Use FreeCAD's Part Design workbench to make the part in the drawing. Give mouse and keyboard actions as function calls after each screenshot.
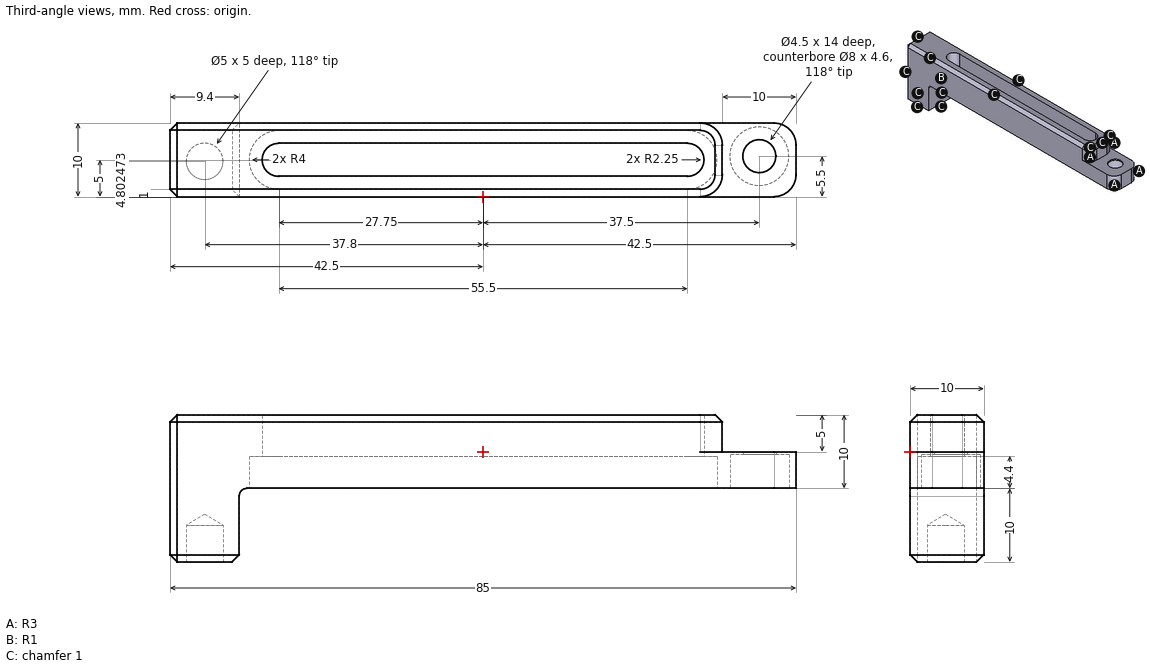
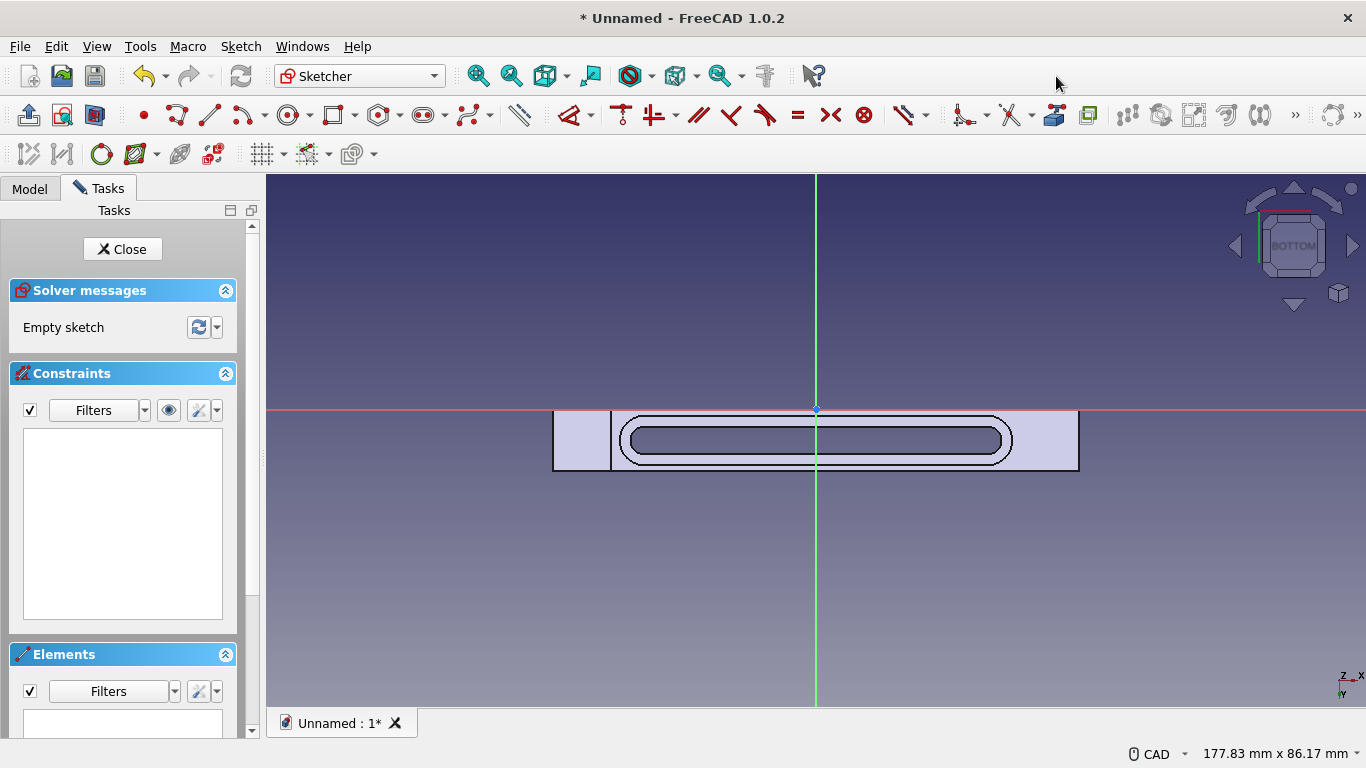
scroll(566, 439, up, 12)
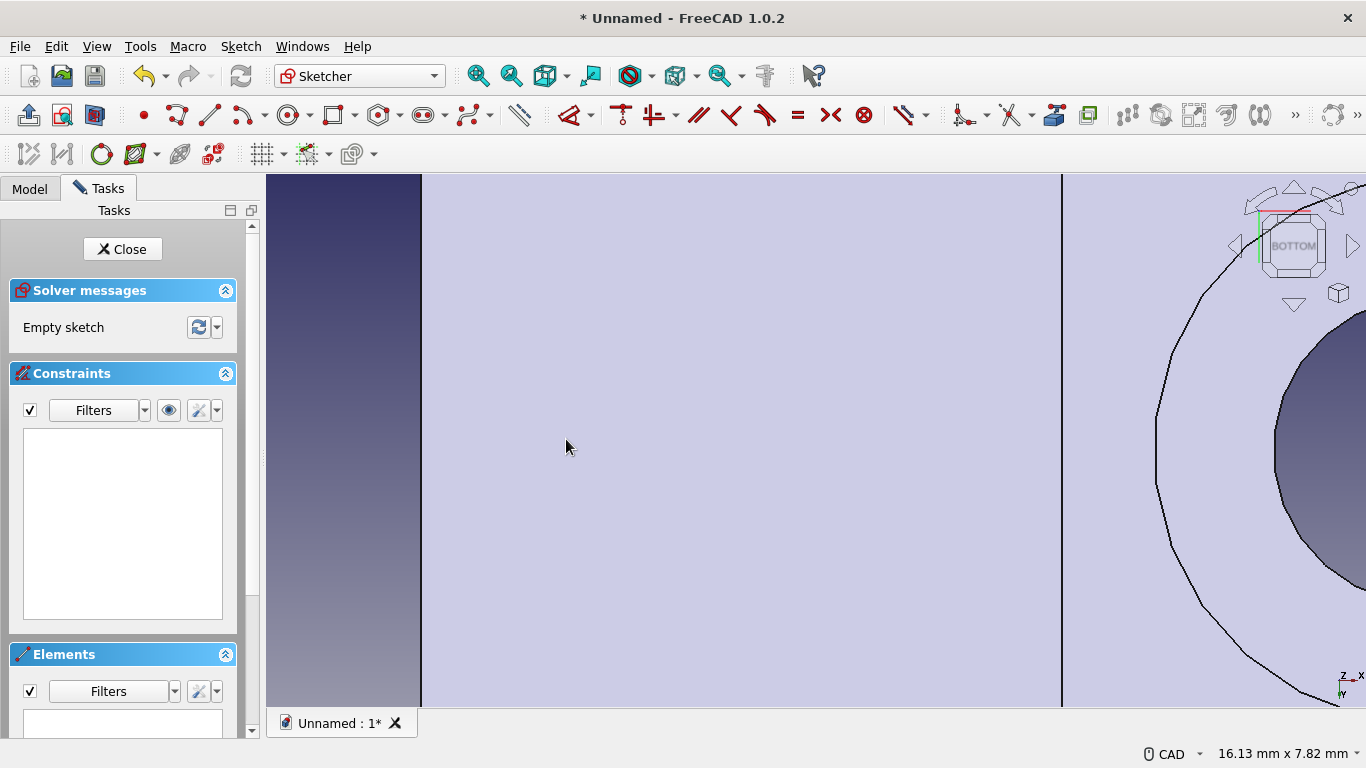
key(g)
key(c)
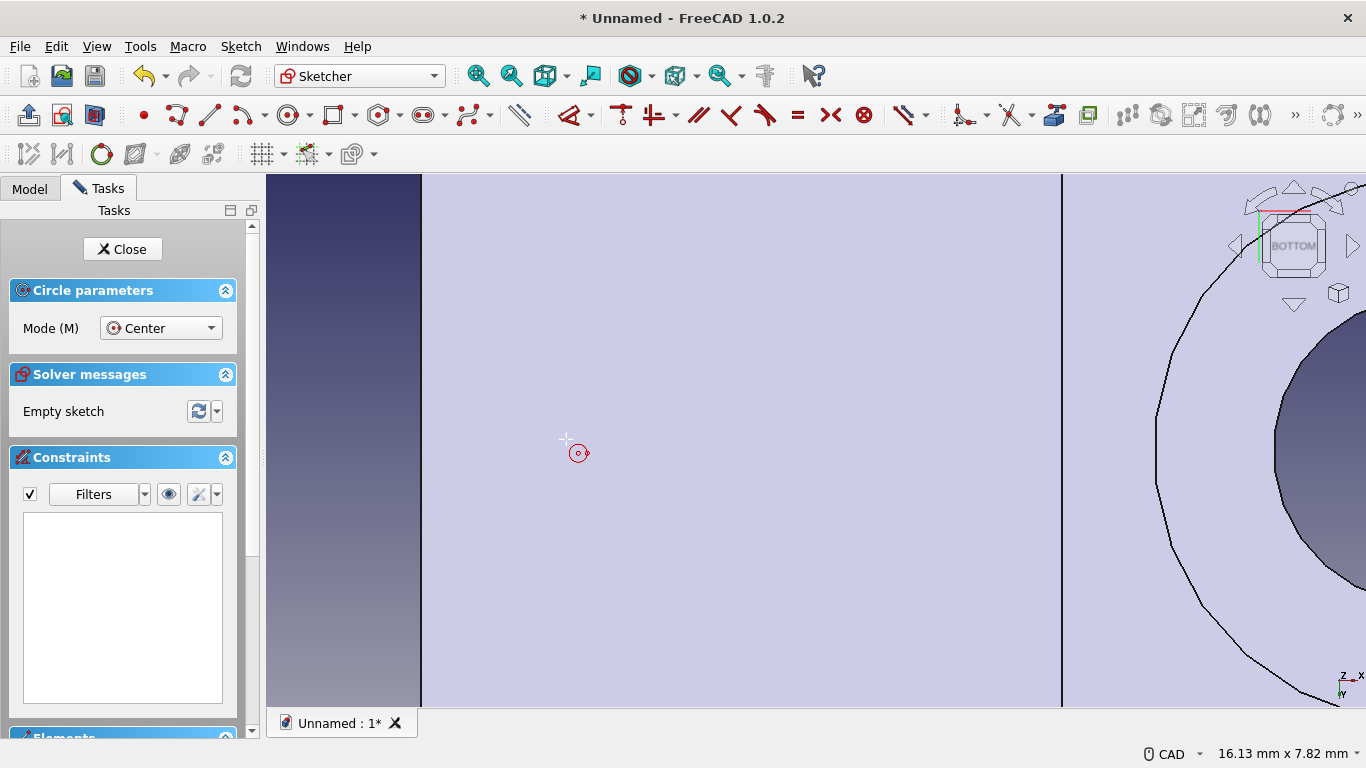
click(742, 437)
click(862, 317)
key(Escape)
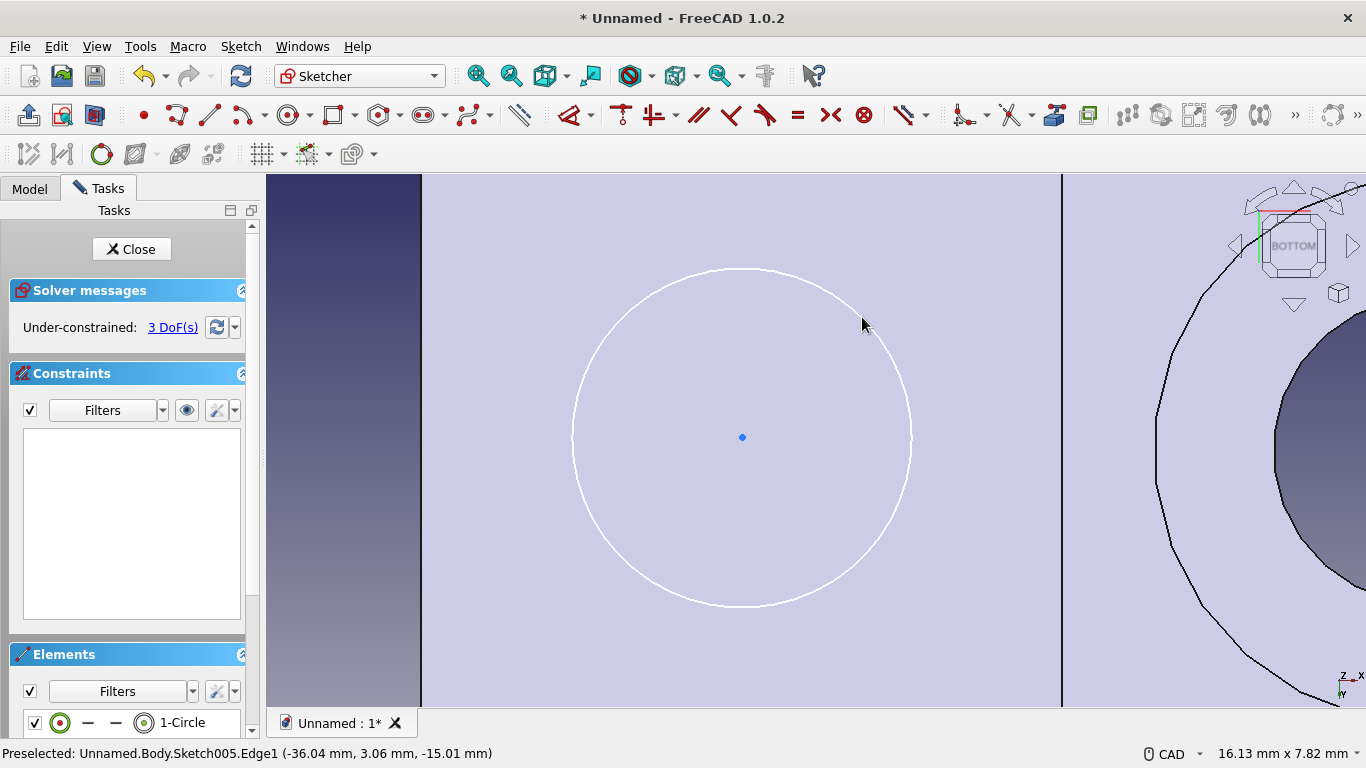
key(d)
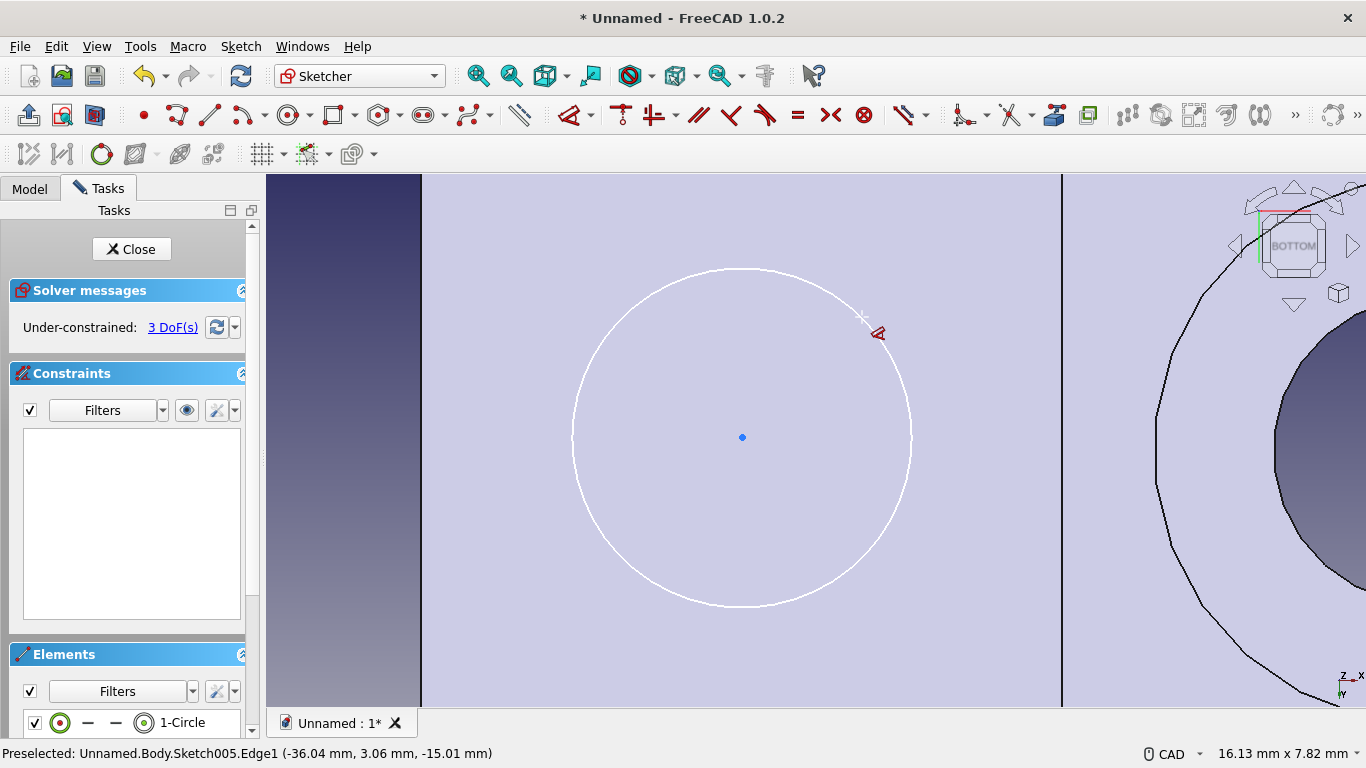
click(862, 318)
click(885, 295)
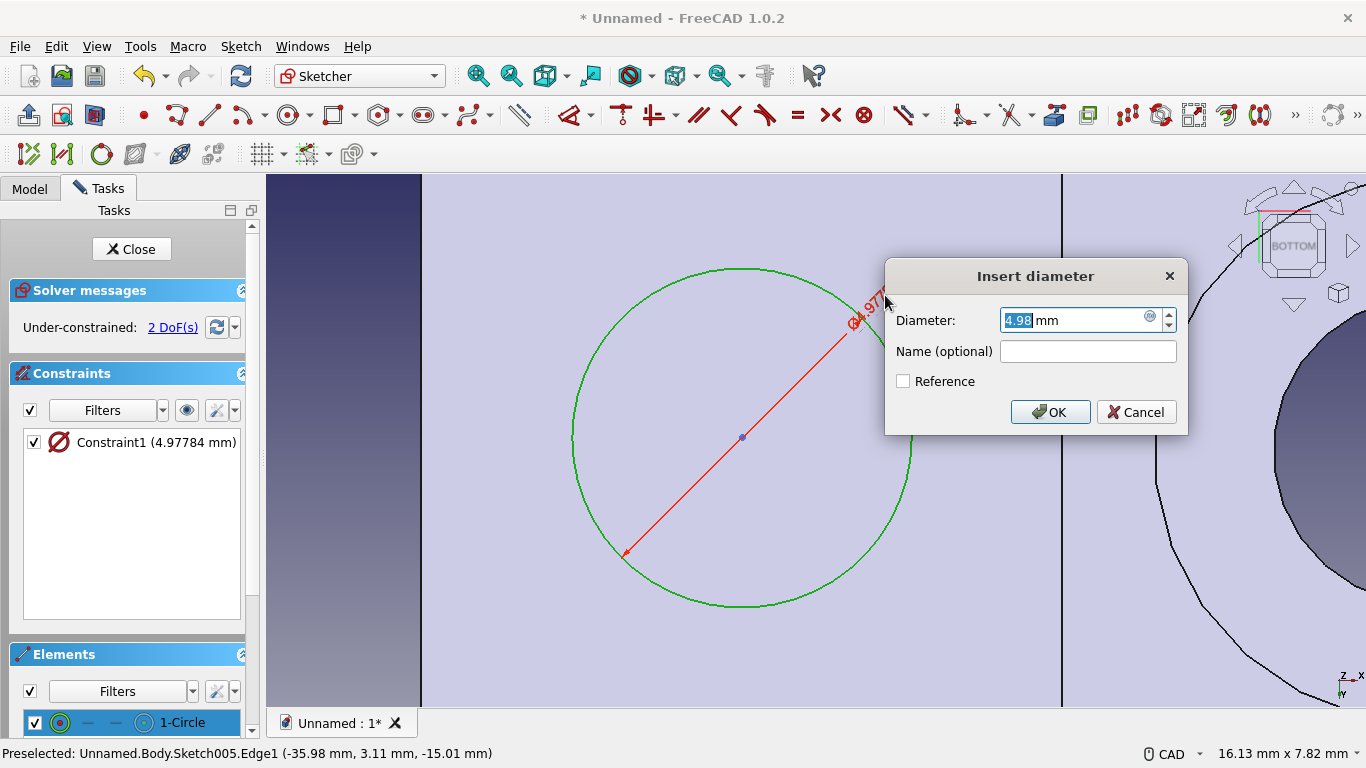
text(5)
key(Return)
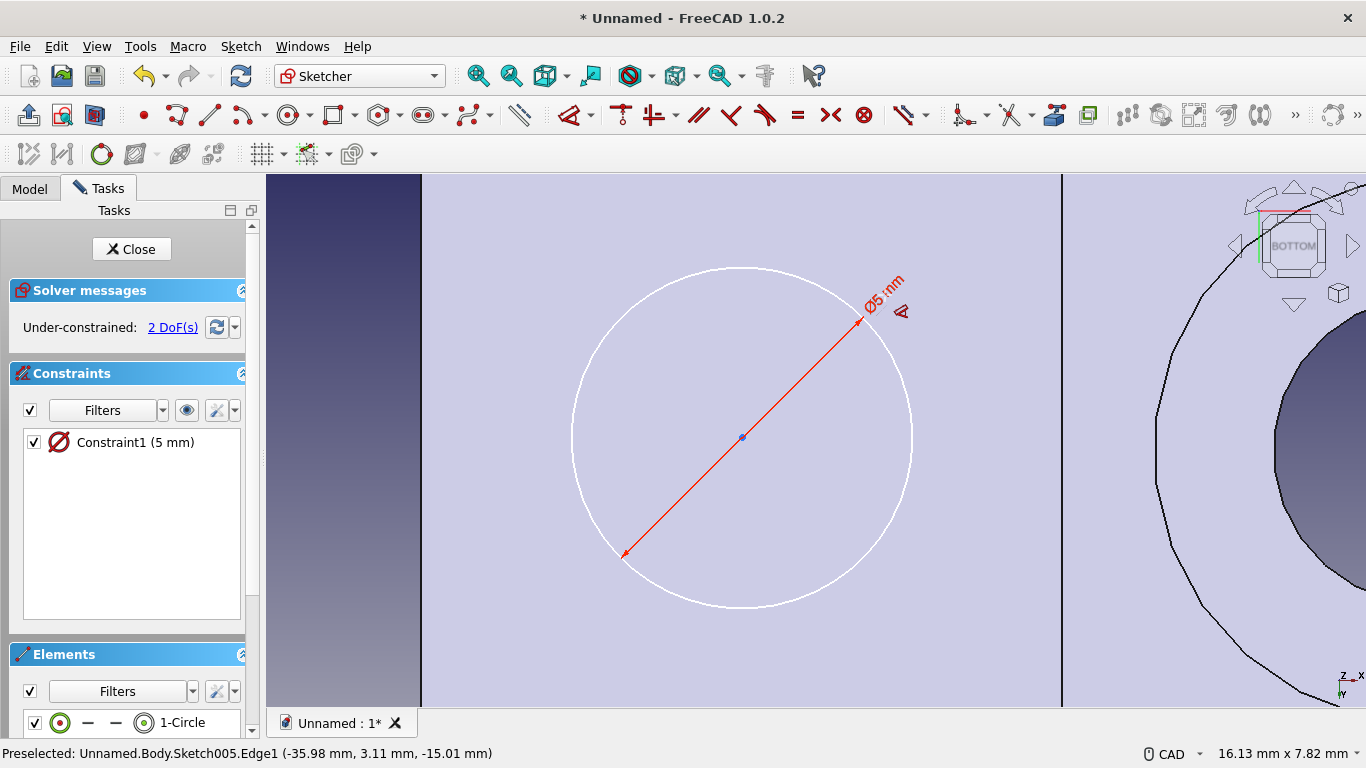
click(742, 438)
click(972, 472)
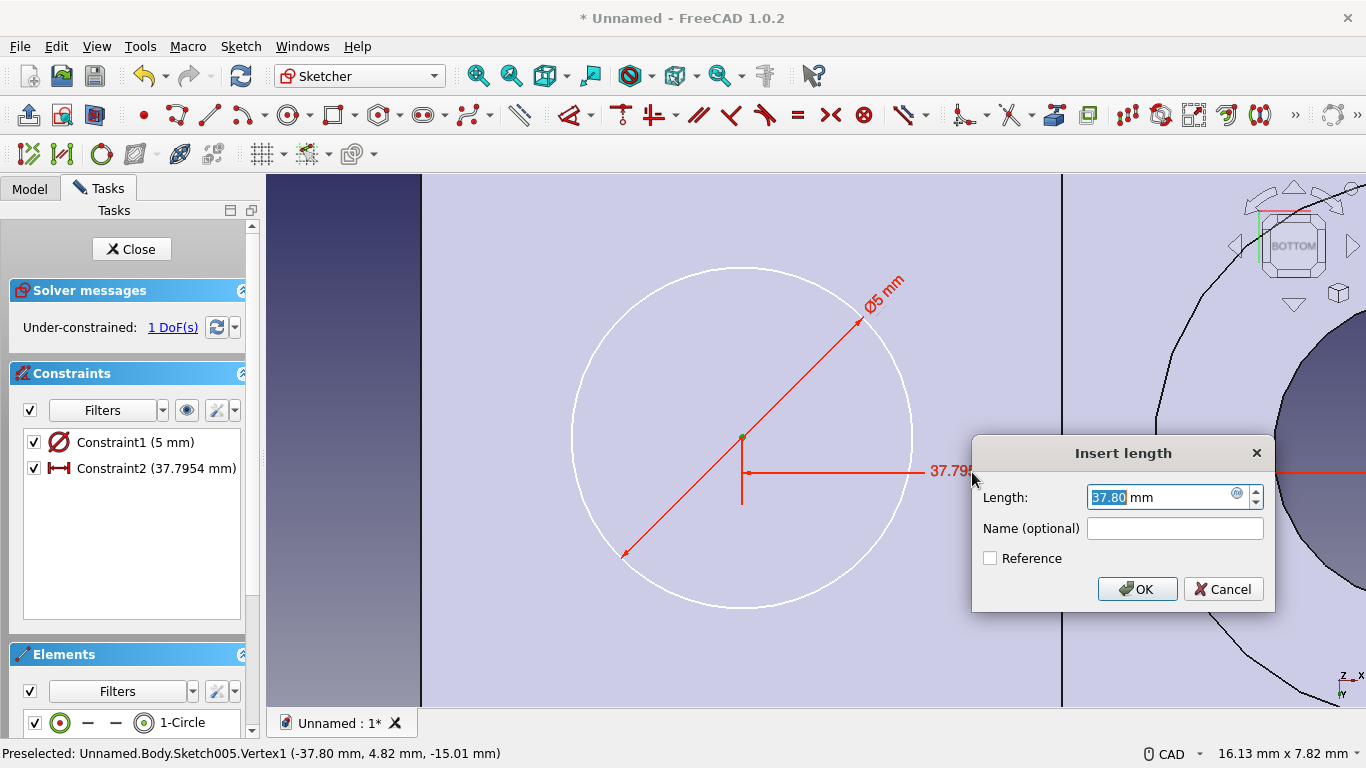
text(37.8)
key(Return)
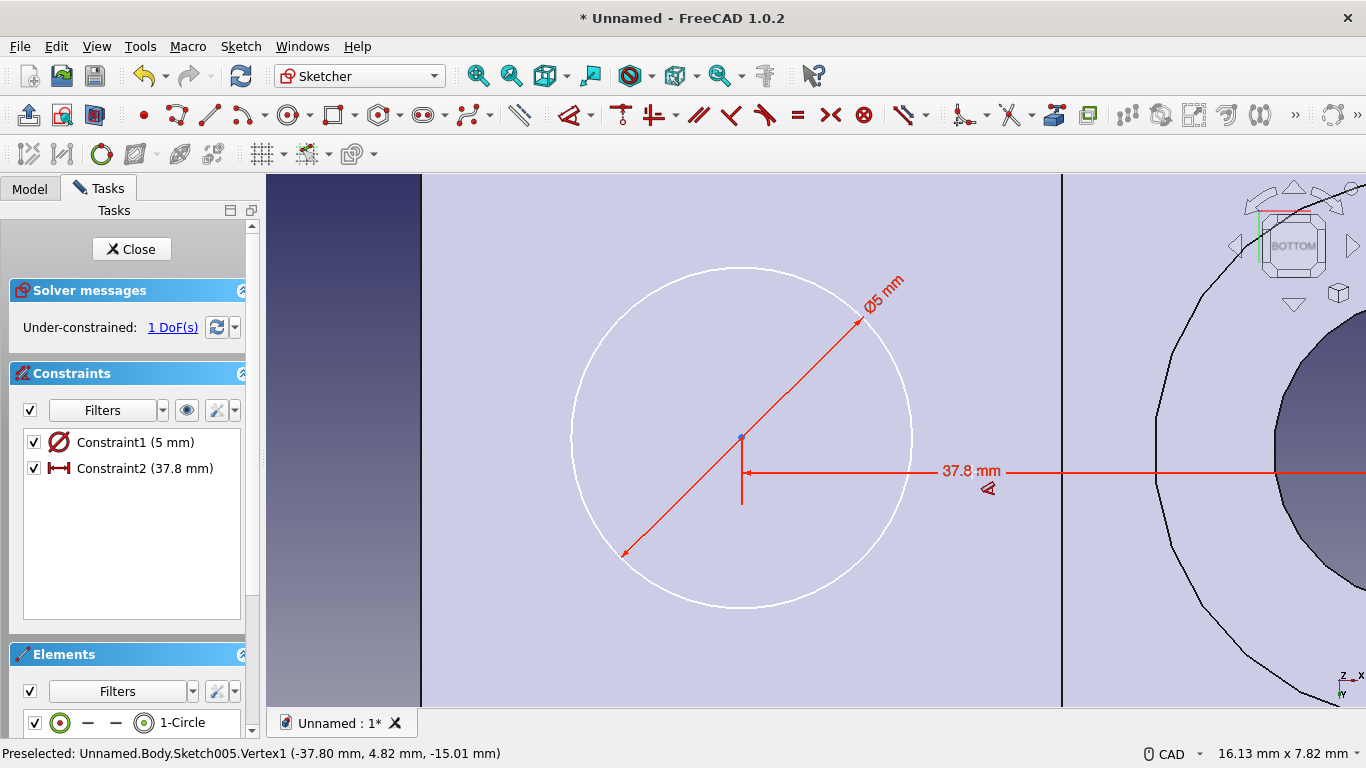
click(742, 438)
click(708, 320)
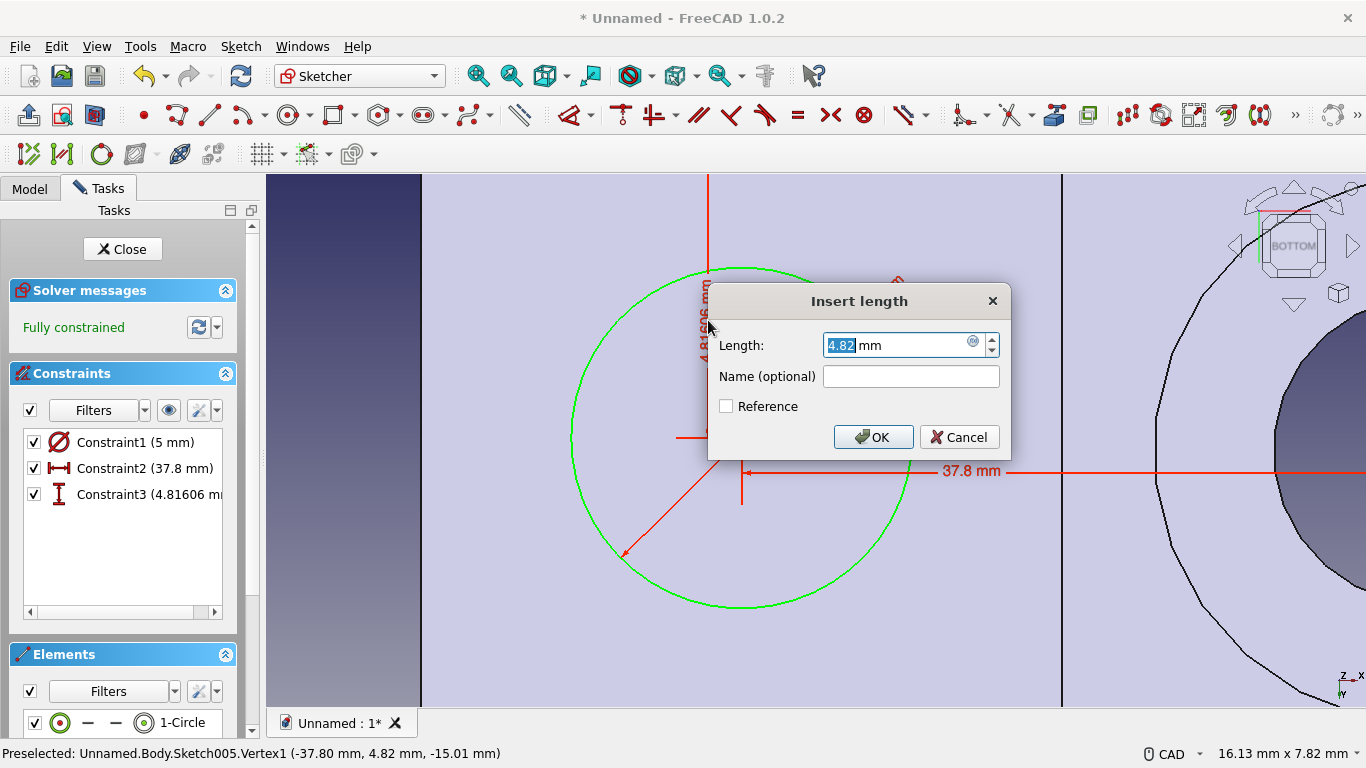
text(4.802473)
key(Return)
key(Escape)